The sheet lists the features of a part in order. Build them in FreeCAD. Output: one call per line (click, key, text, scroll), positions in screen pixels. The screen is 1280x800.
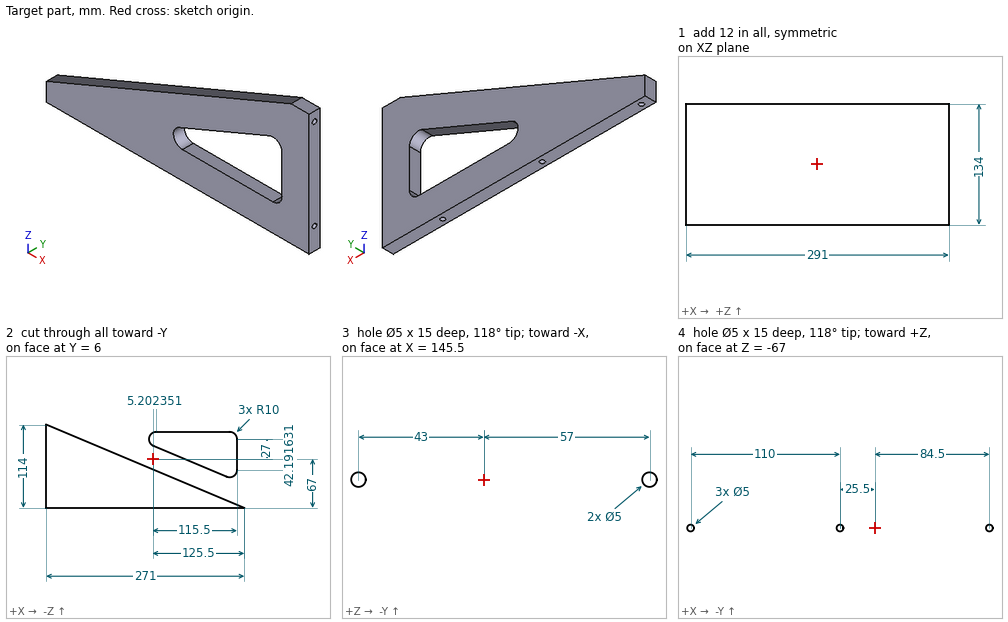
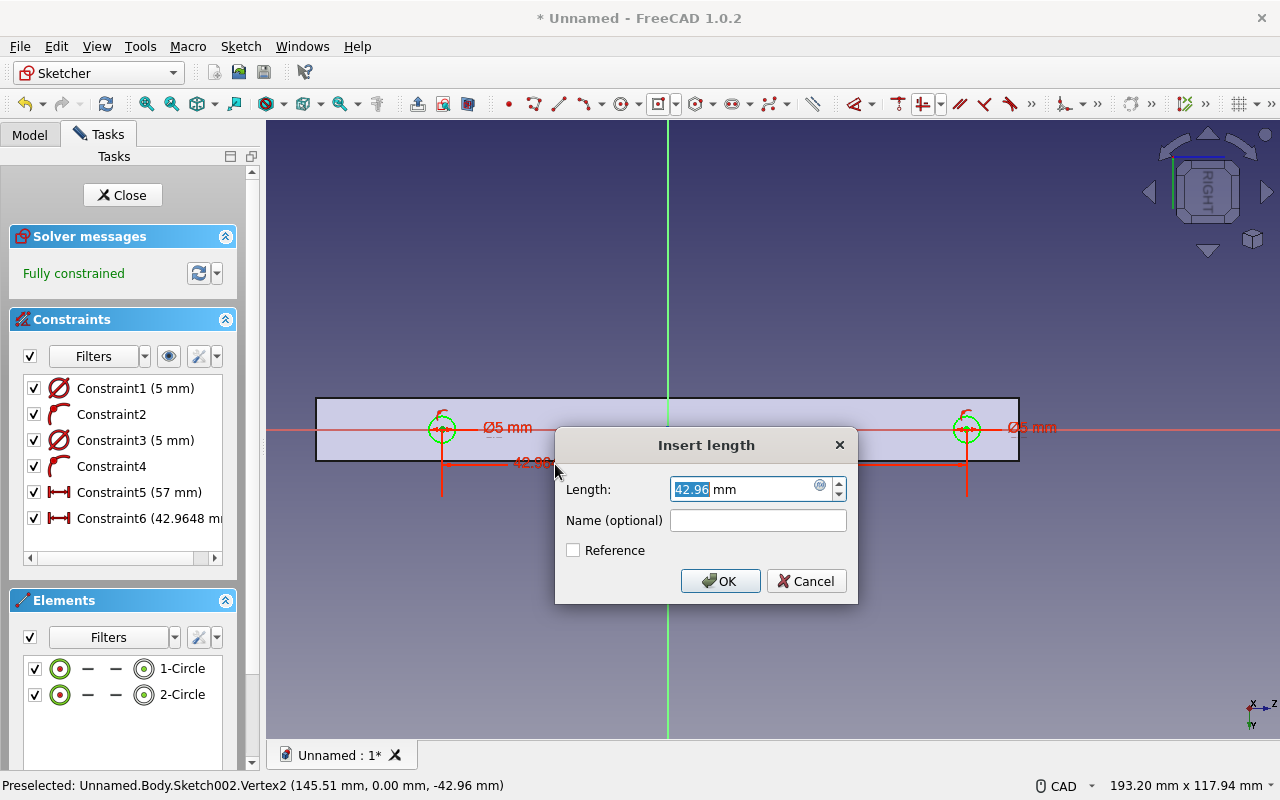
text(43)
key(Return)
key(Escape)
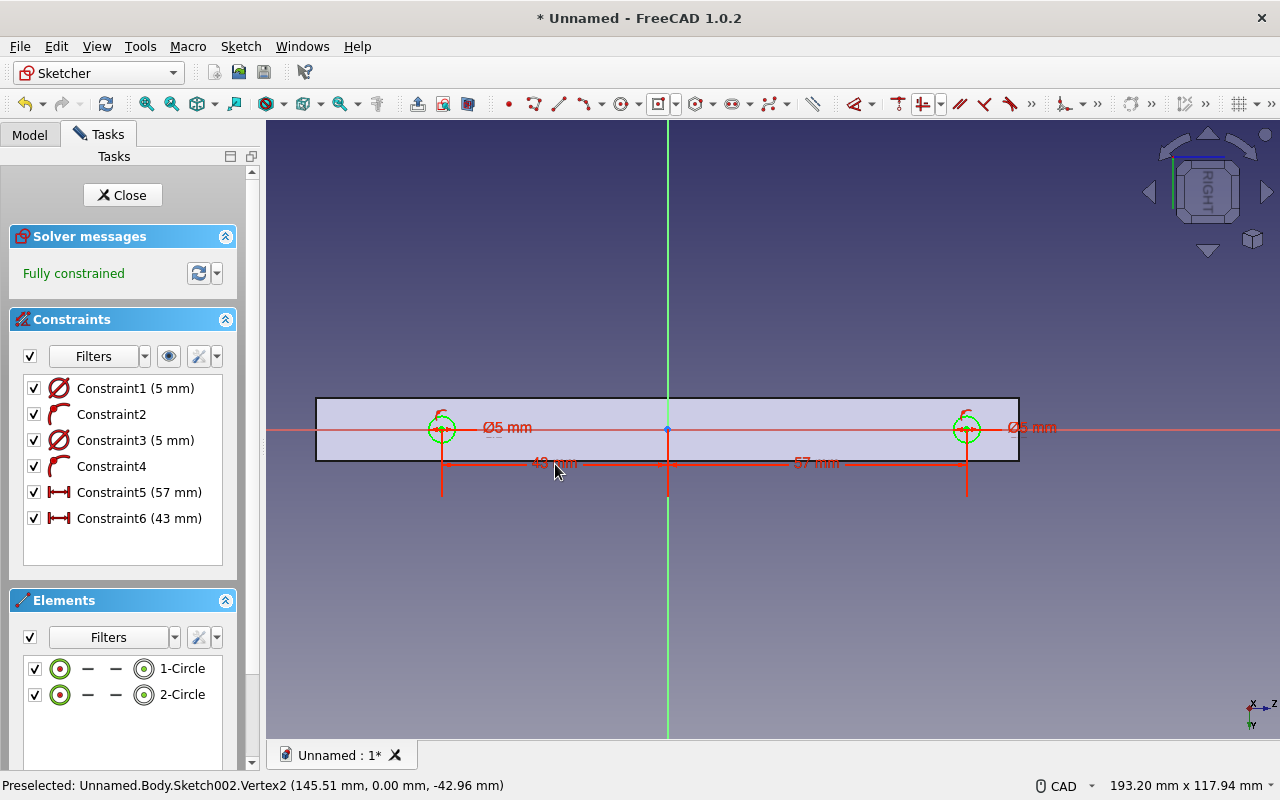
click(123, 195)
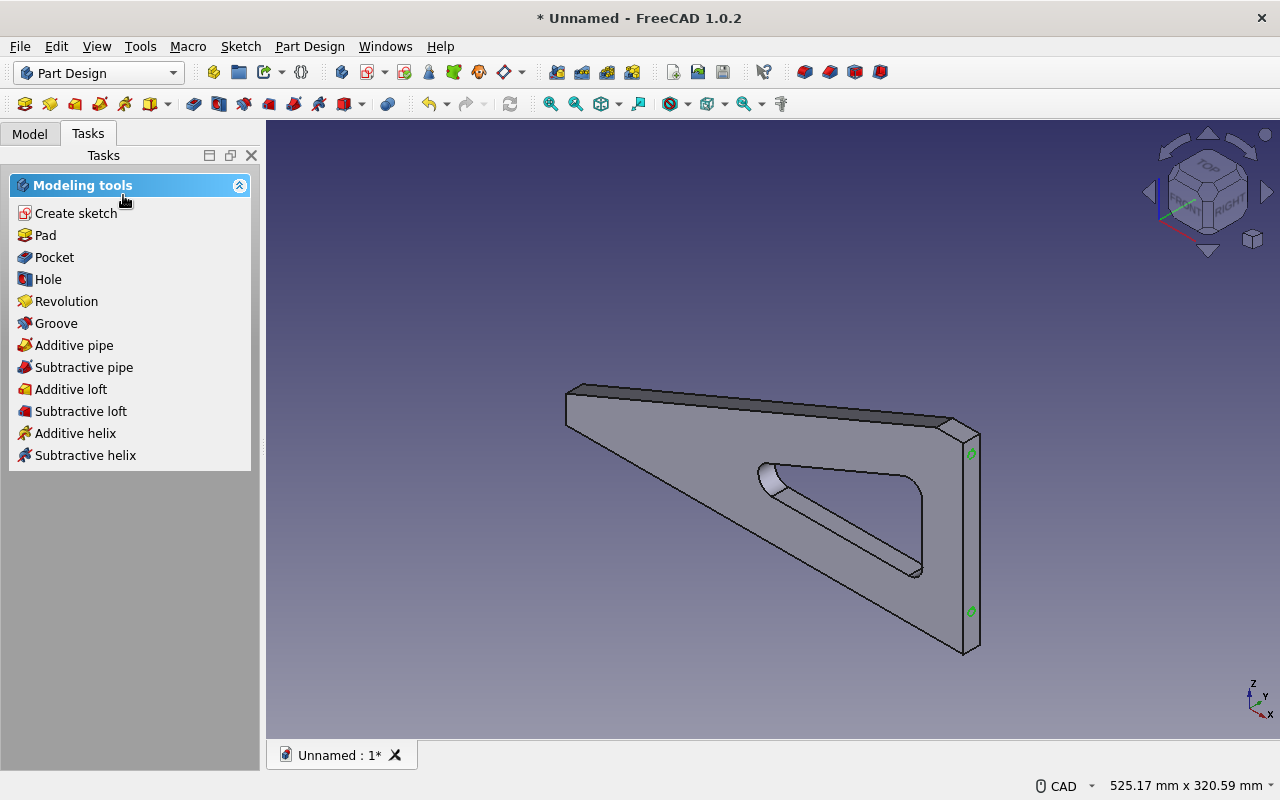
click(219, 104)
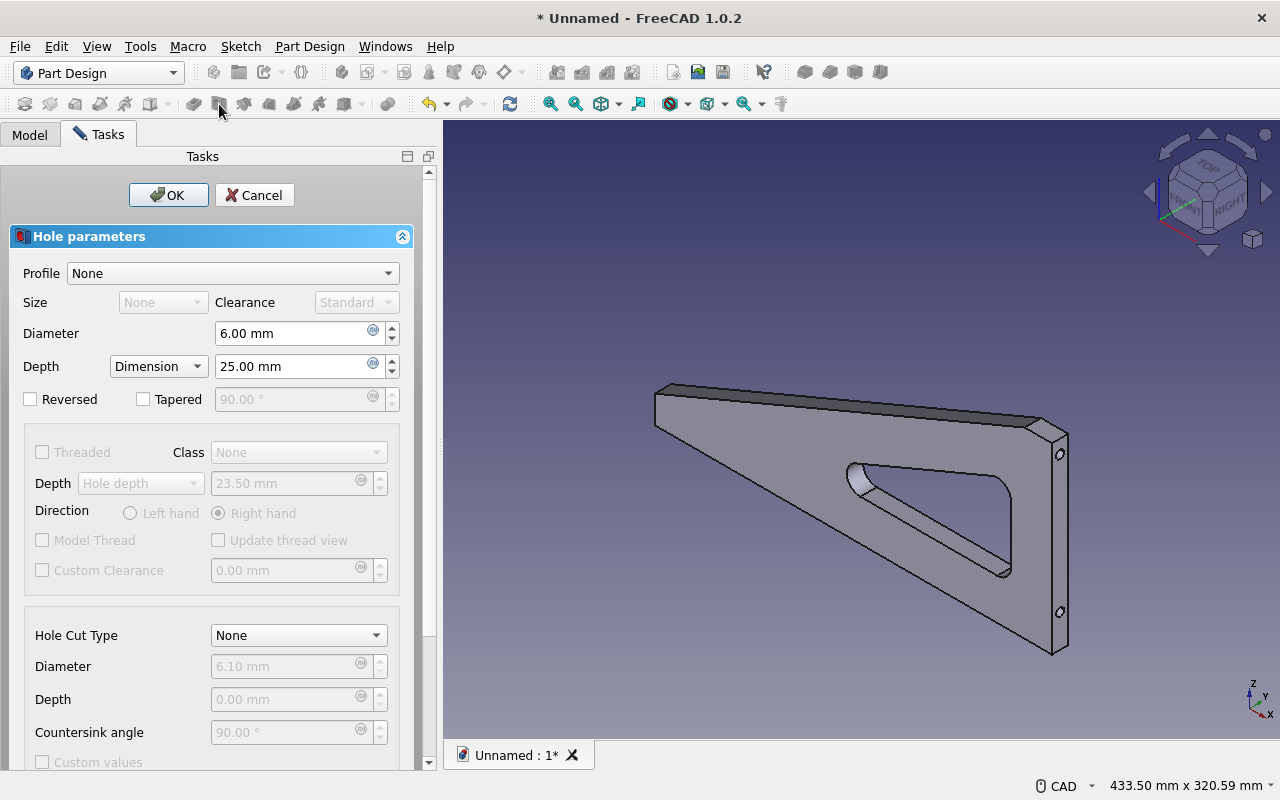
triple_click(300, 334)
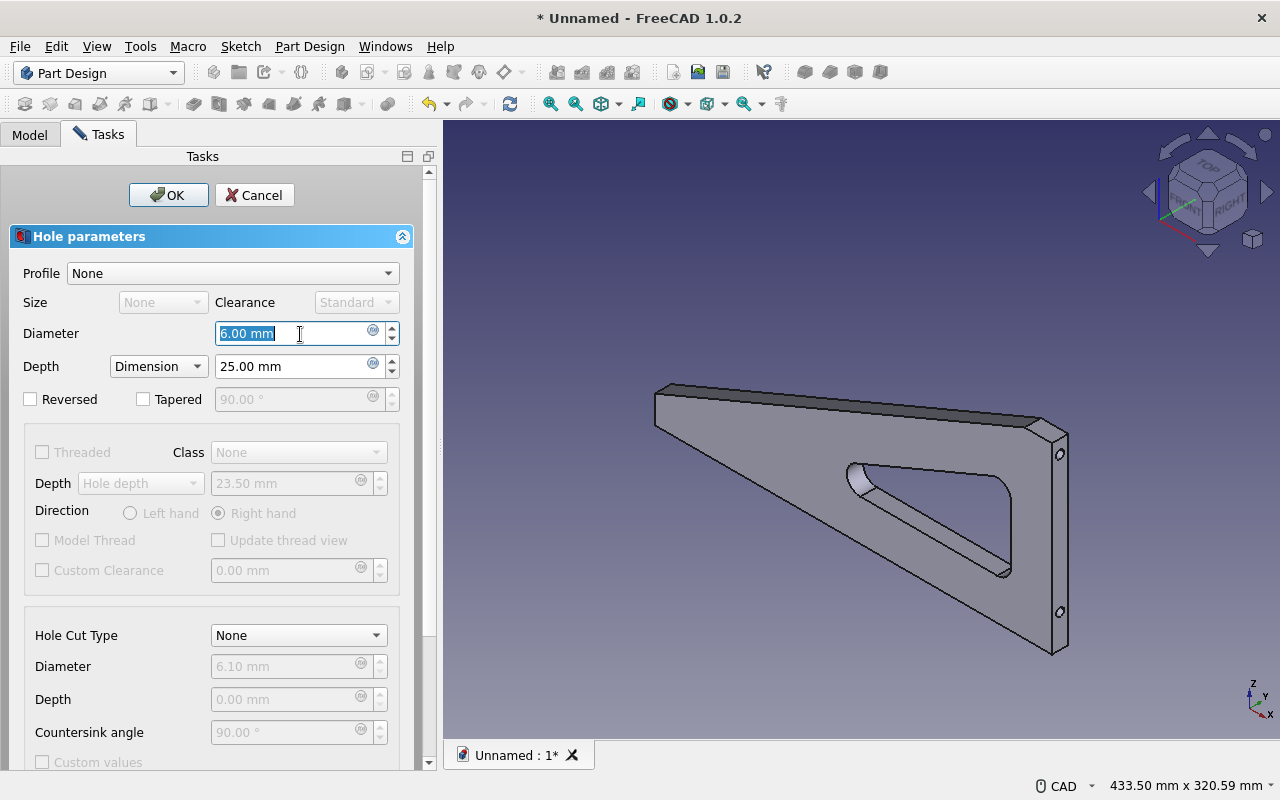
text(5)
key(Tab)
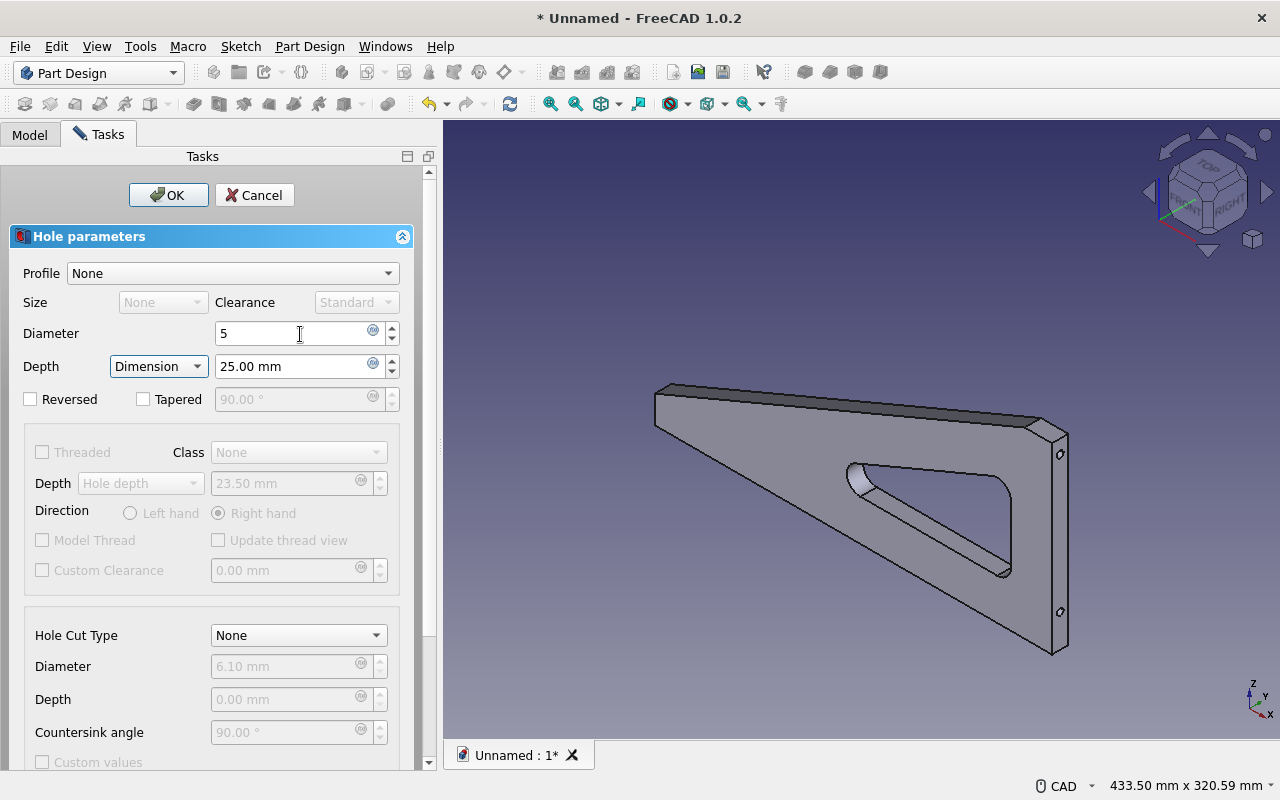
triple_click(300, 366)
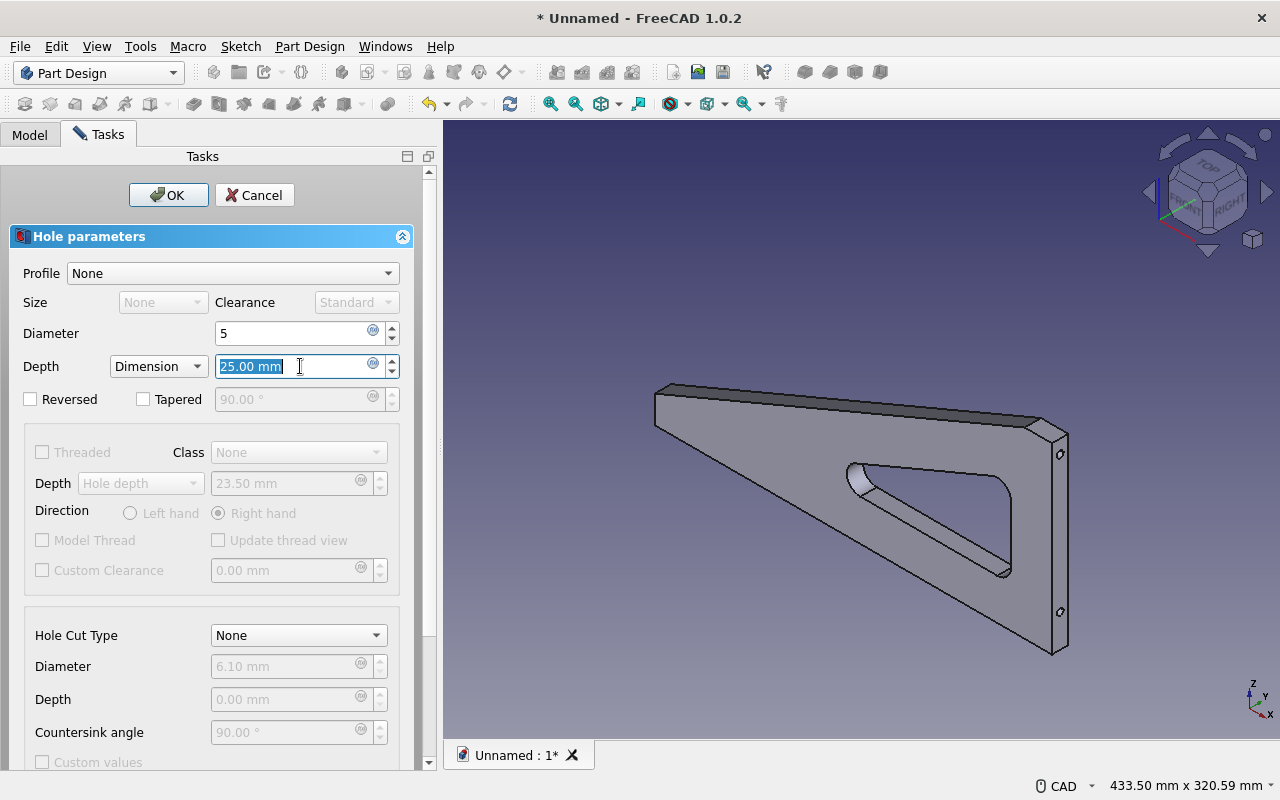
text(15)
key(Tab)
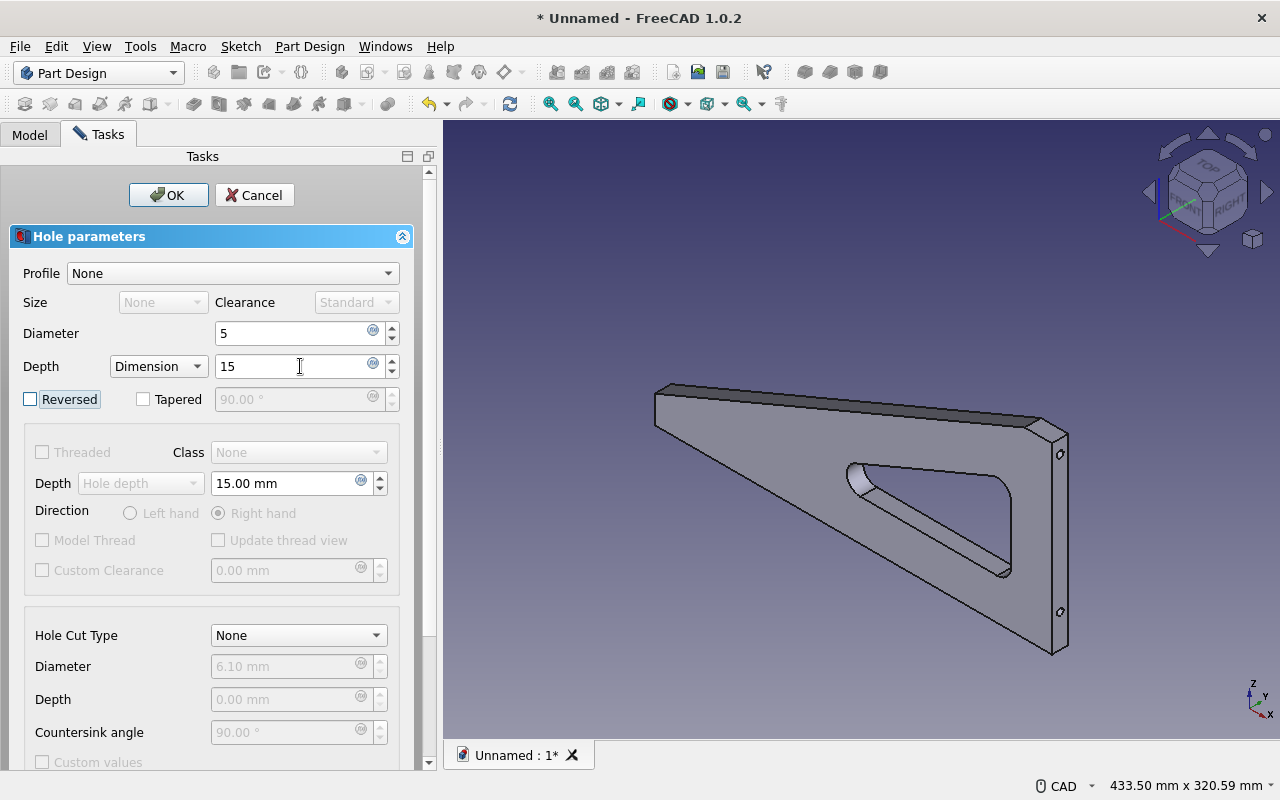
click(169, 195)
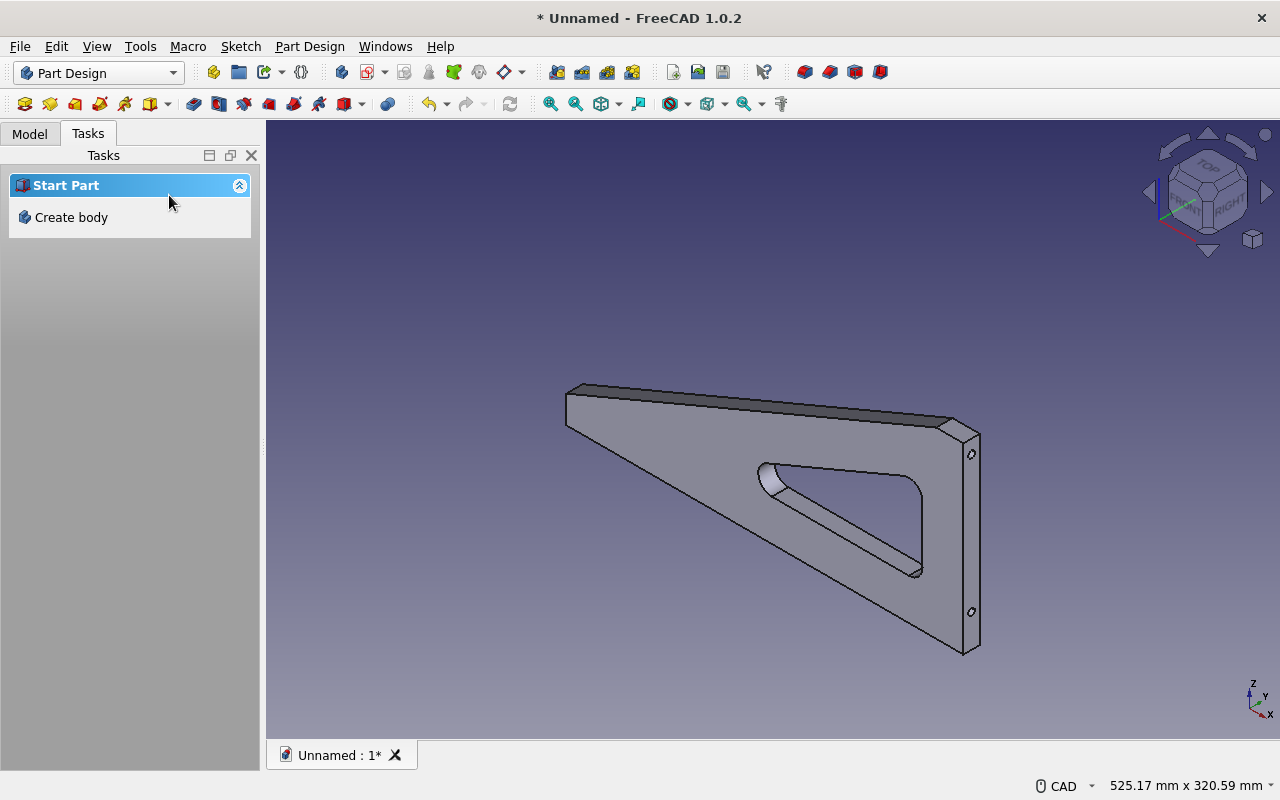
key(5)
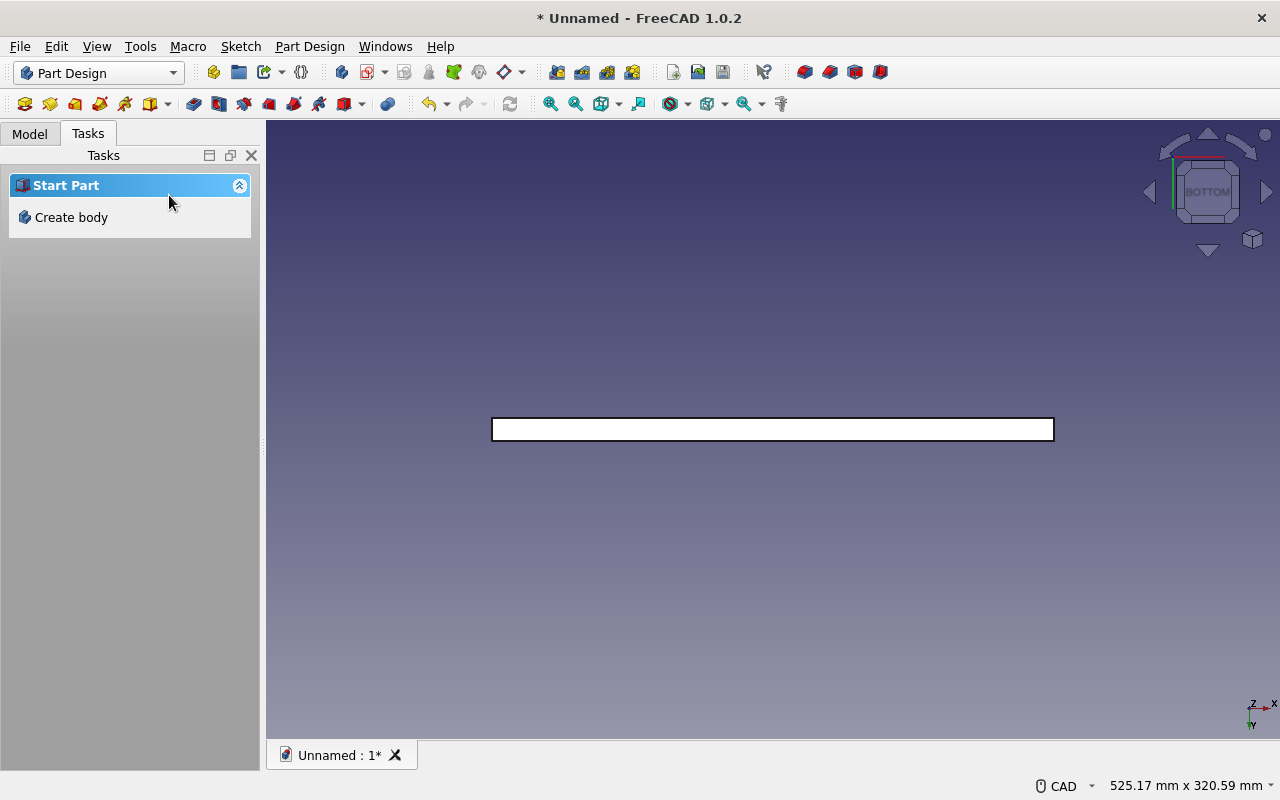
click(1014, 429)